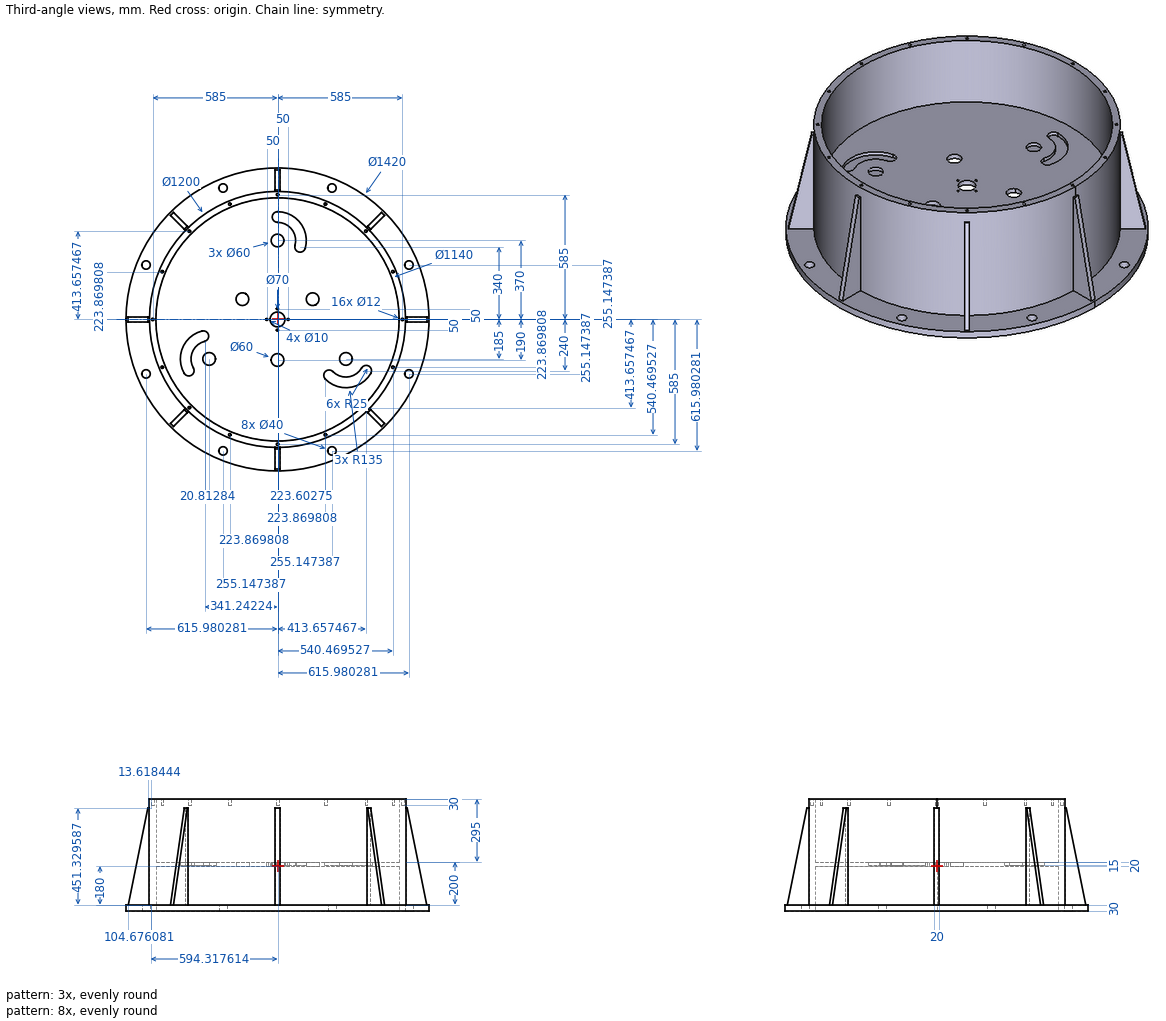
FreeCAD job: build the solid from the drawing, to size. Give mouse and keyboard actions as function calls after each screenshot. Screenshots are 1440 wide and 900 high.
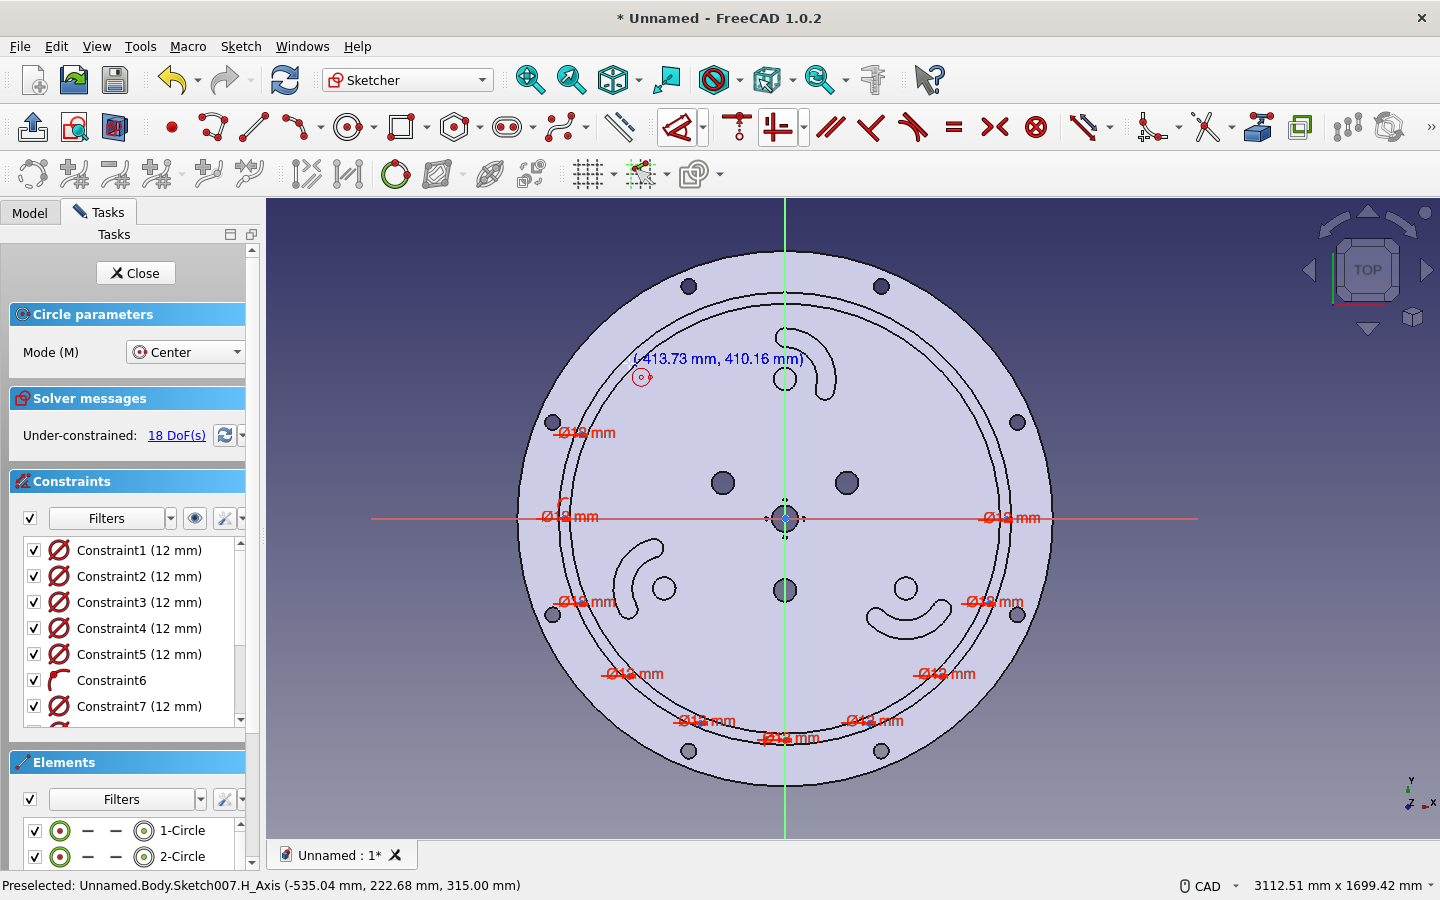
click(629, 363)
move(631, 361)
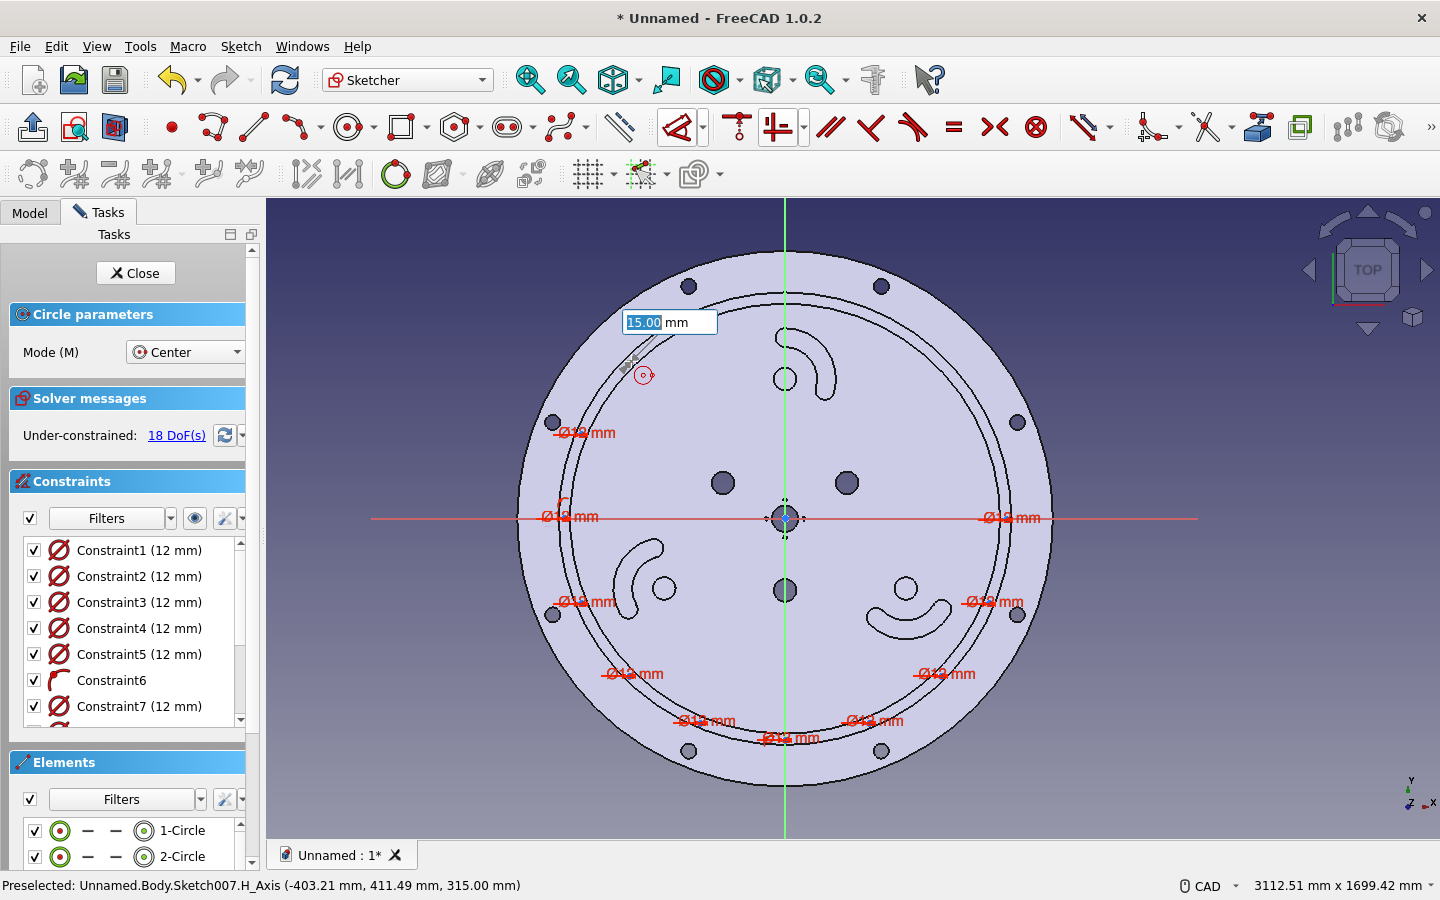
text(12)
key(Return)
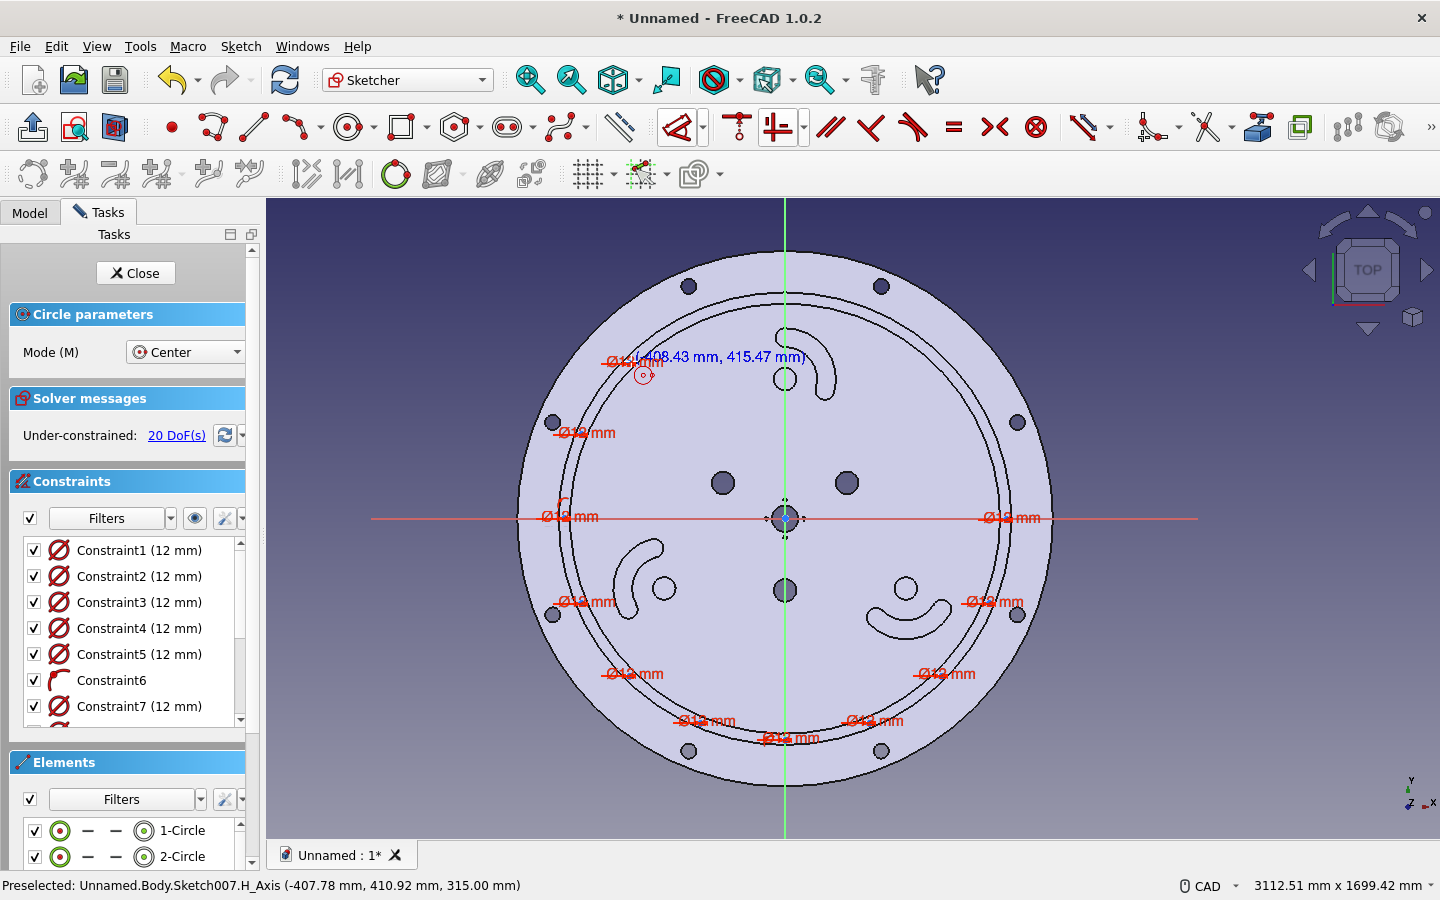
scroll(701, 315, up, 12)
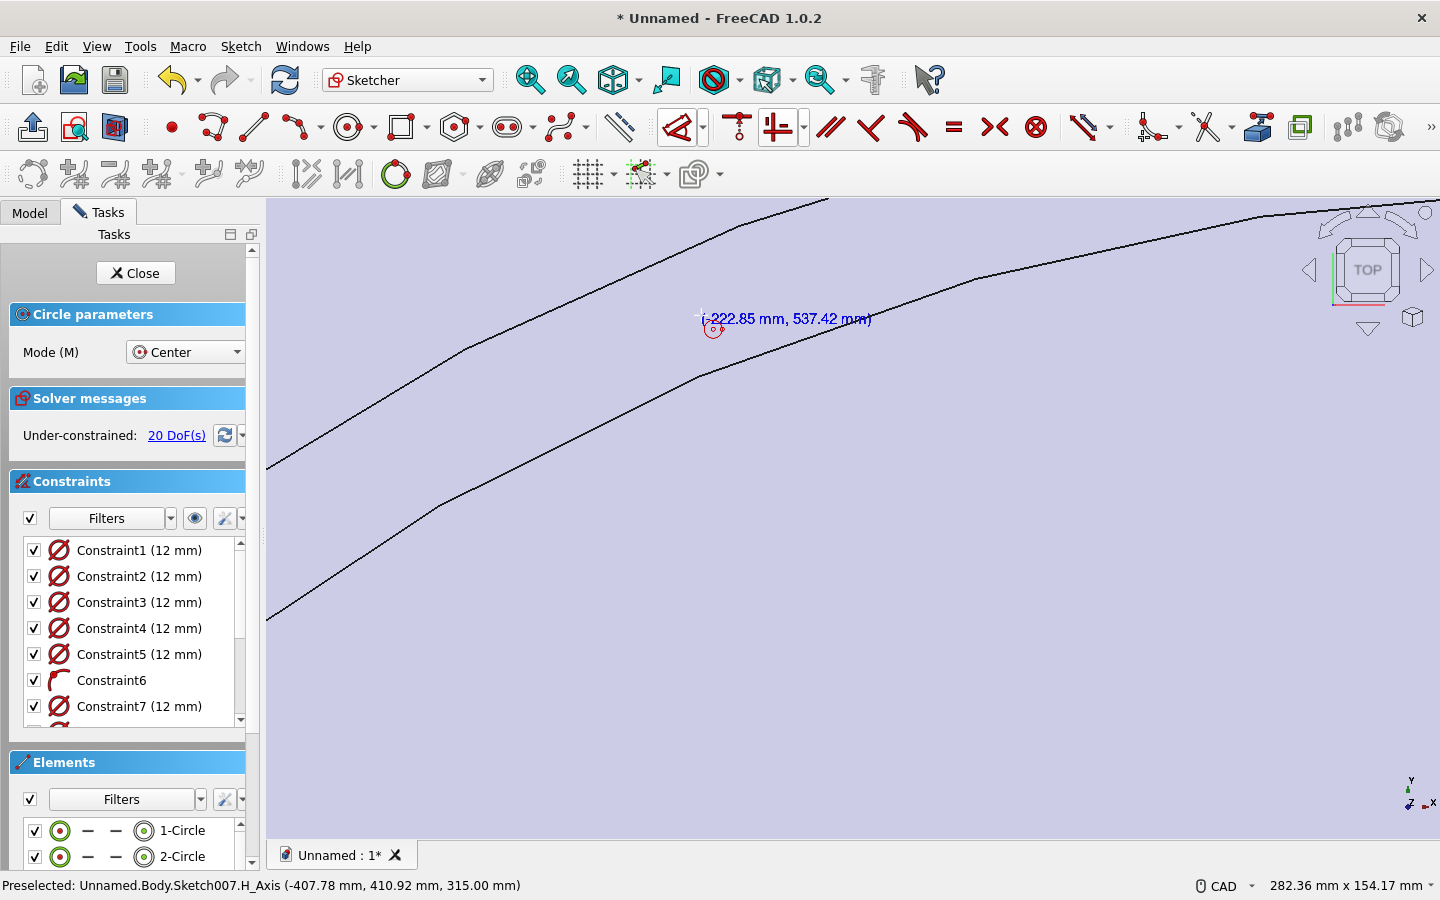
scroll(701, 315, down, 12)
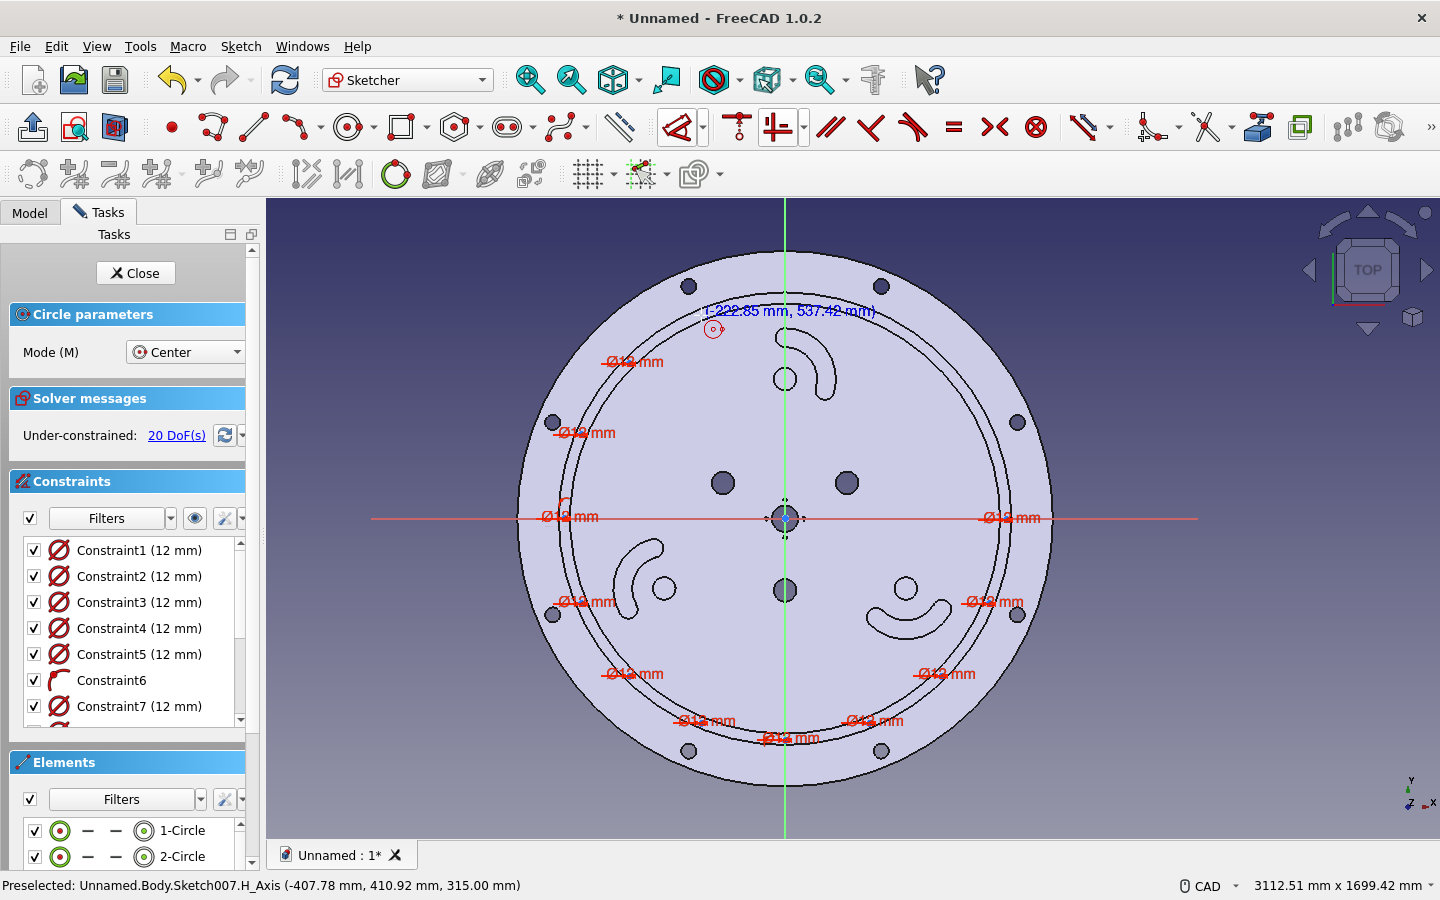
click(701, 315)
move(702, 313)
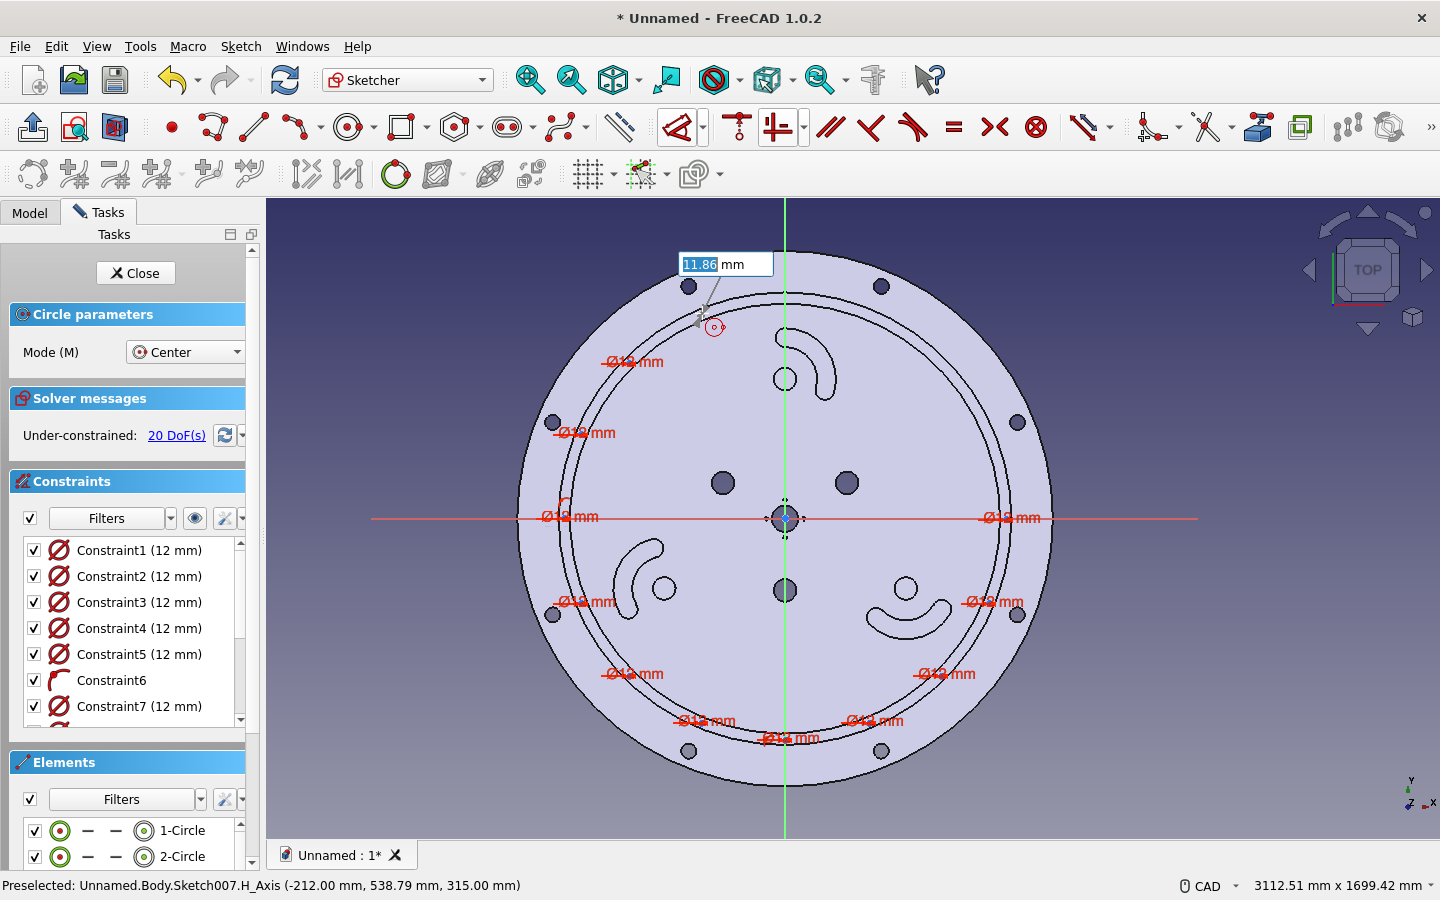
text(12)
key(Return)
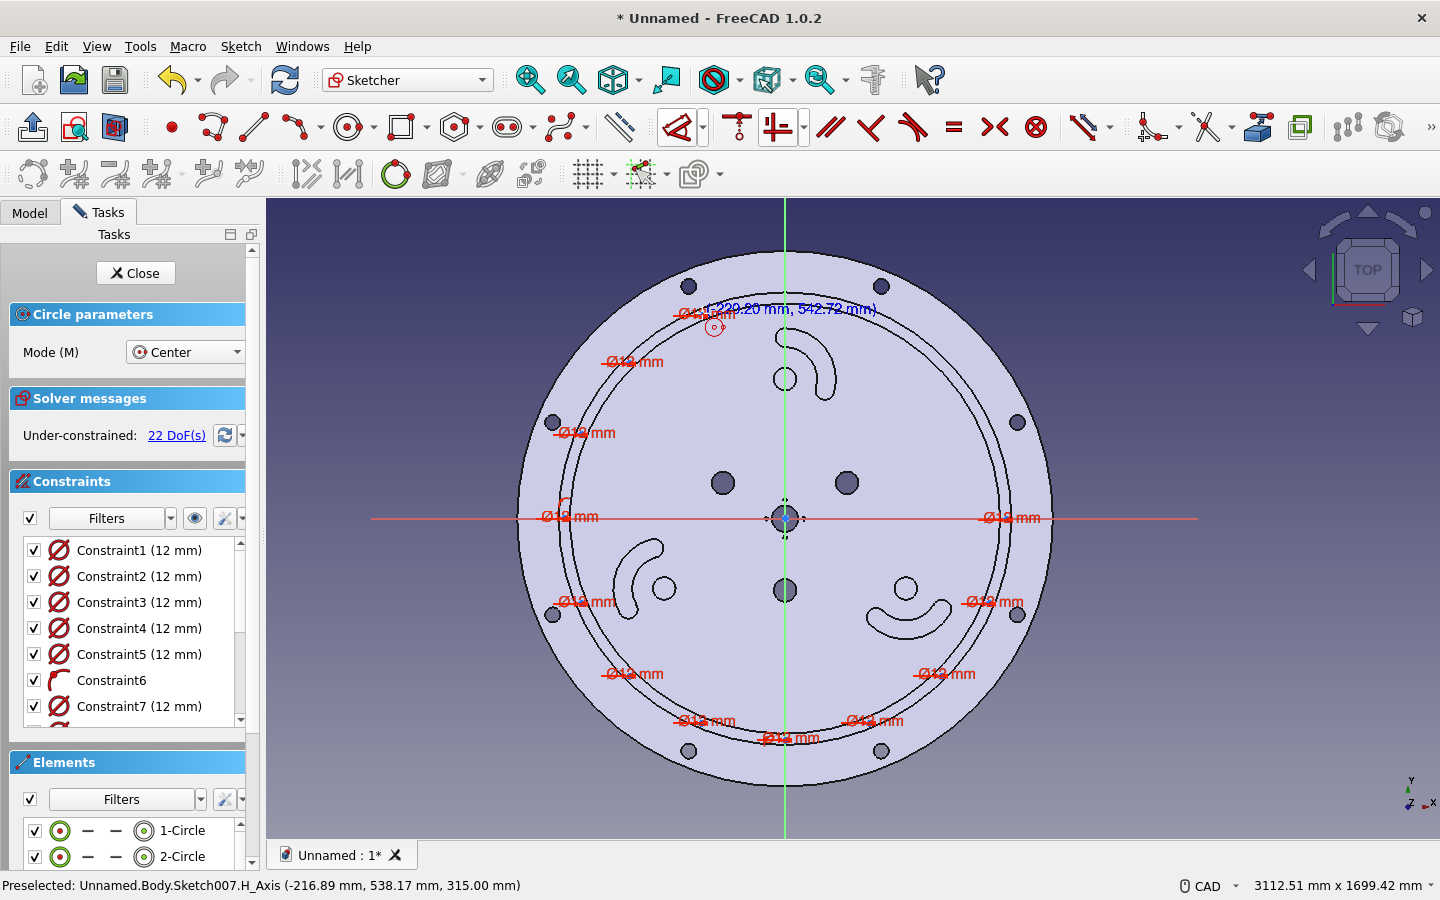
scroll(785, 298, up, 12)